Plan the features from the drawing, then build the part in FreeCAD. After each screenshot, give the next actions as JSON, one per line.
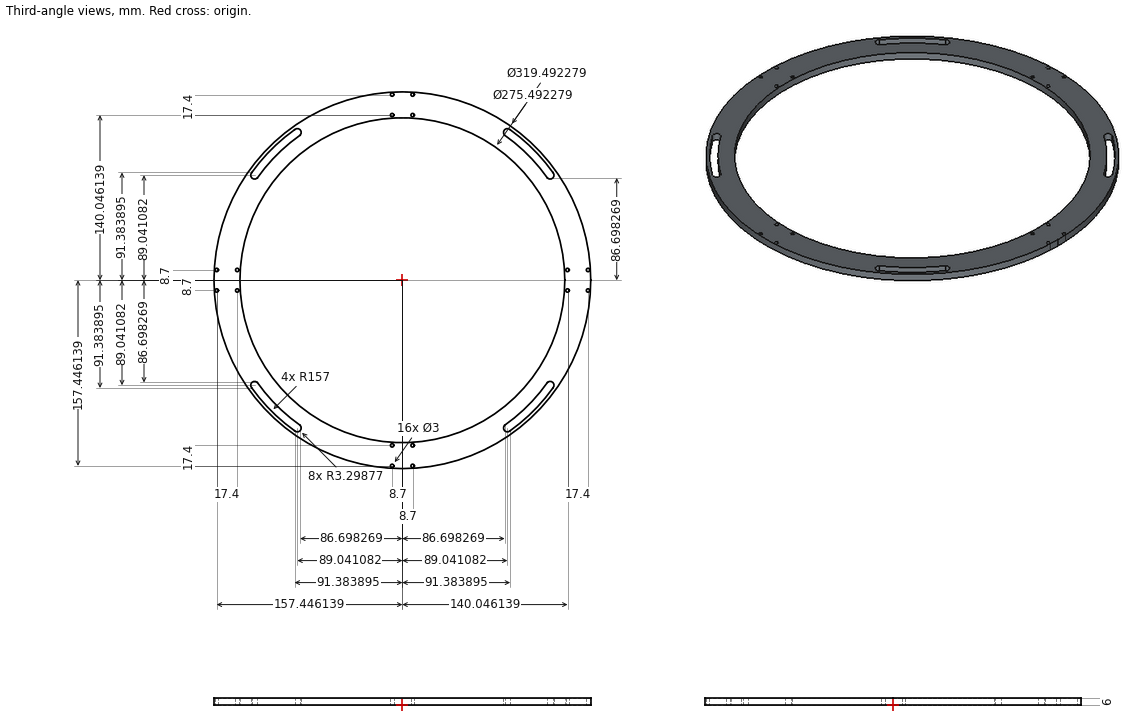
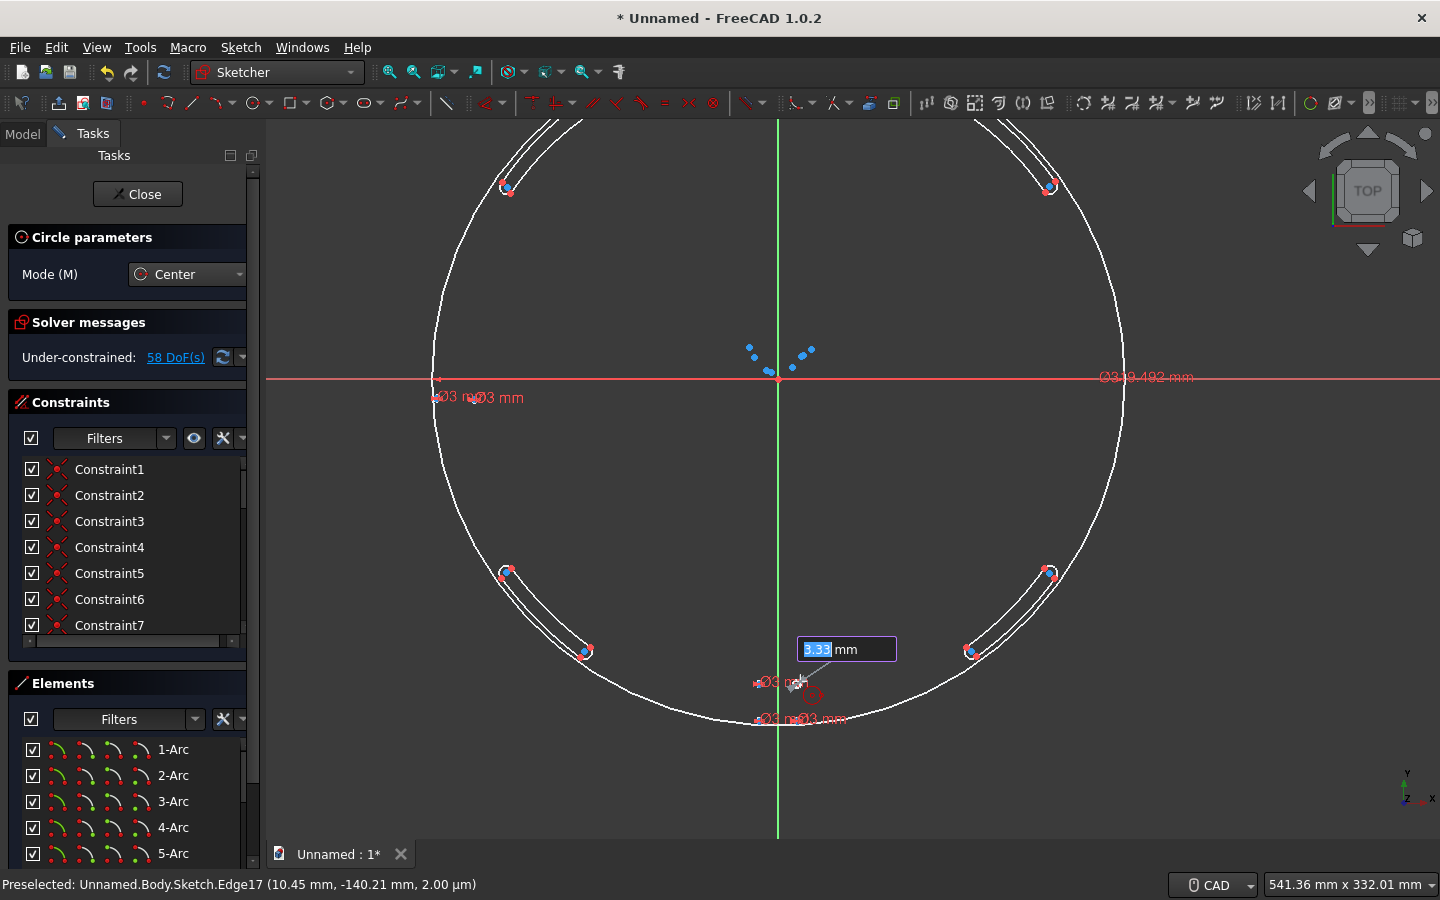
{"action": "type", "text": "3"}
{"action": "key", "text": "Return"}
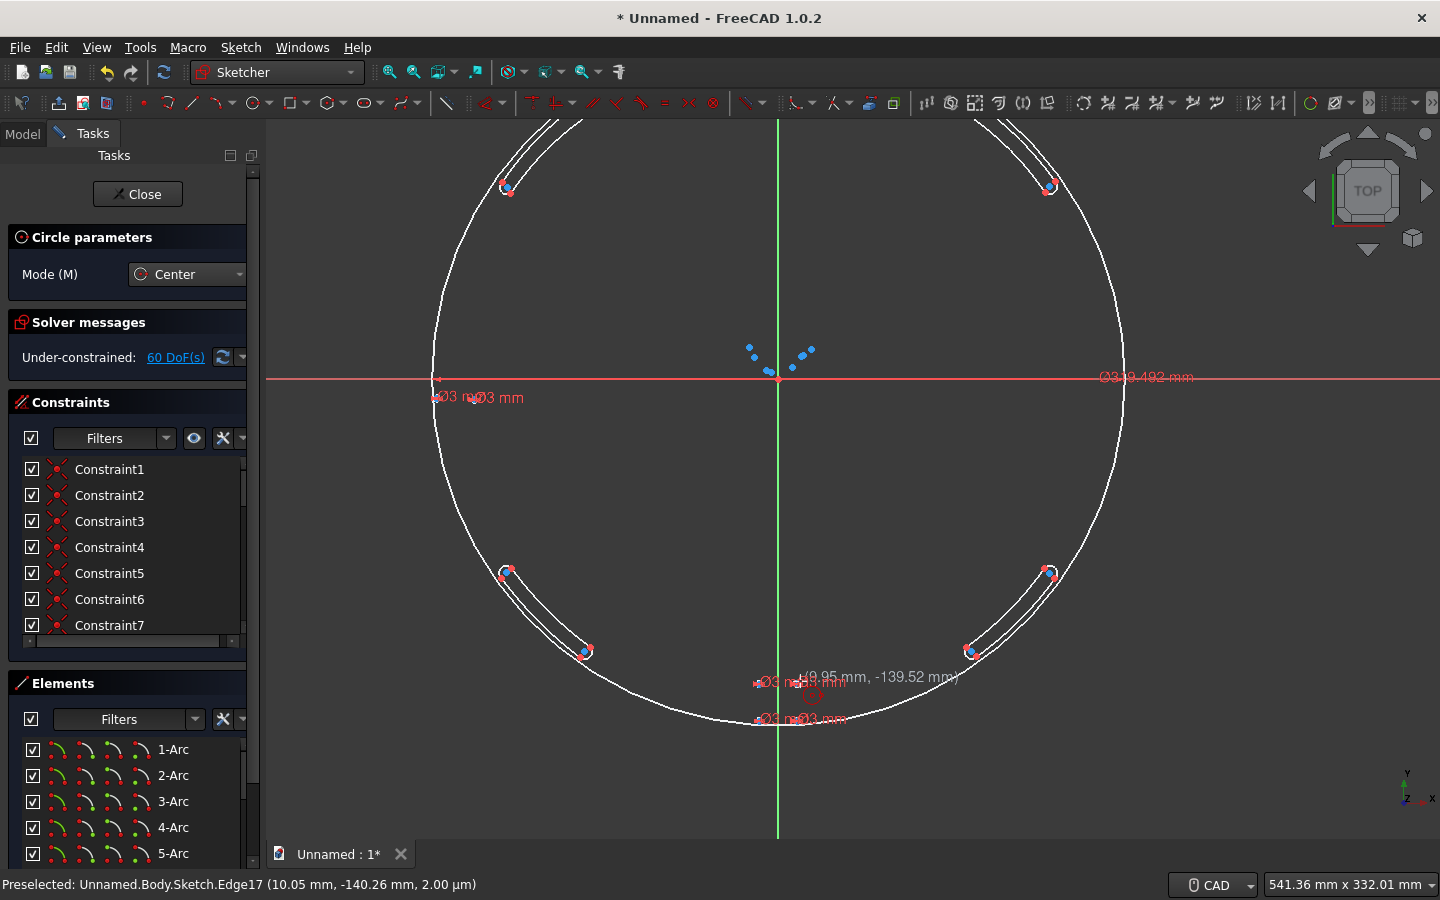
{"action": "scroll", "coordinate": [1082, 398], "scroll_direction": "up", "scroll_amount": 10}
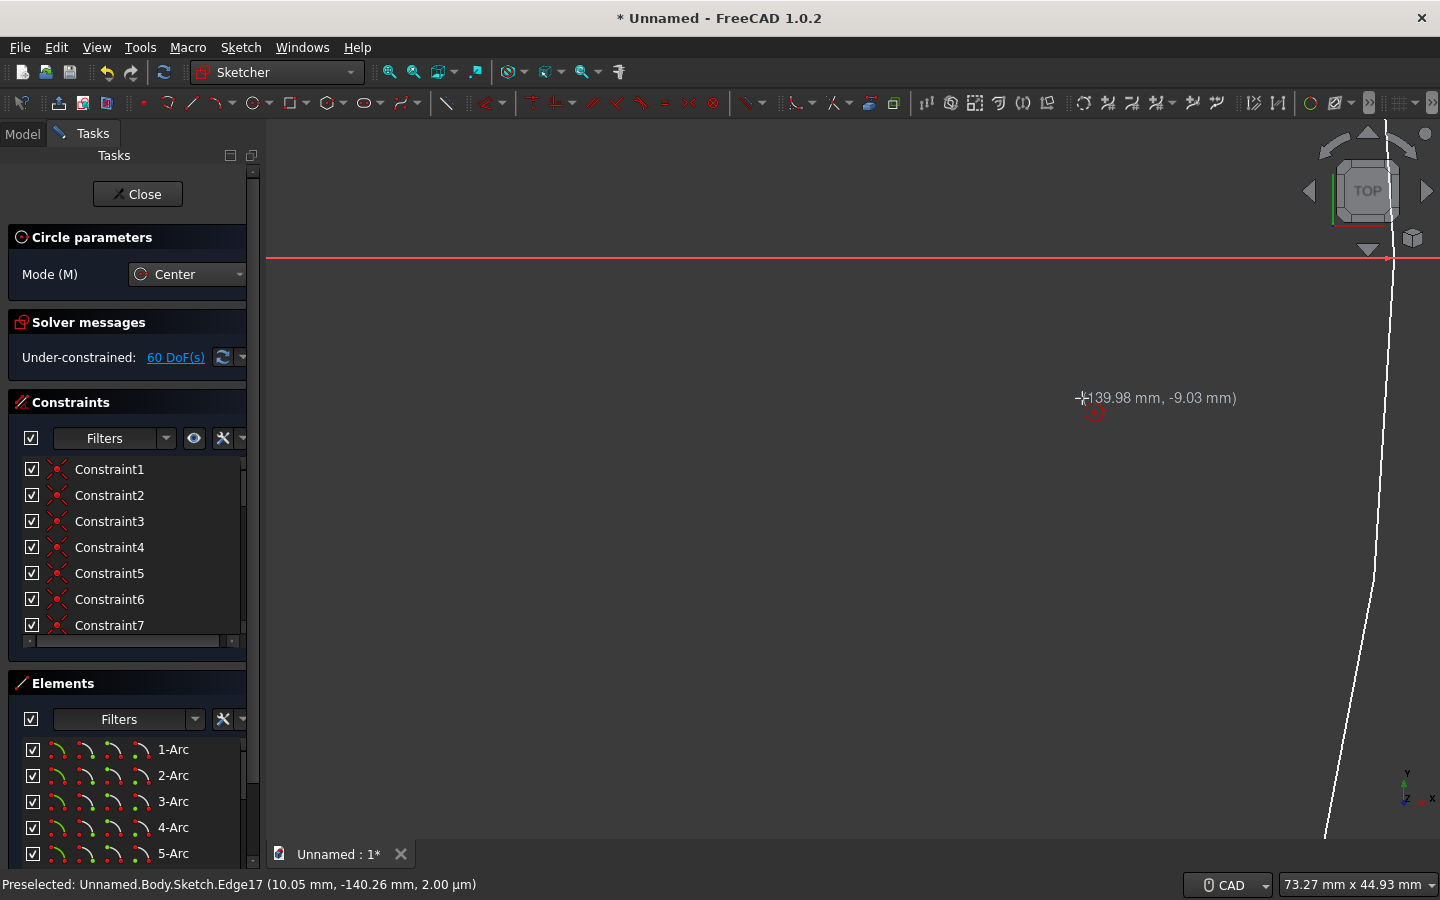
{"action": "scroll", "coordinate": [979, 501], "scroll_direction": "down", "scroll_amount": 12}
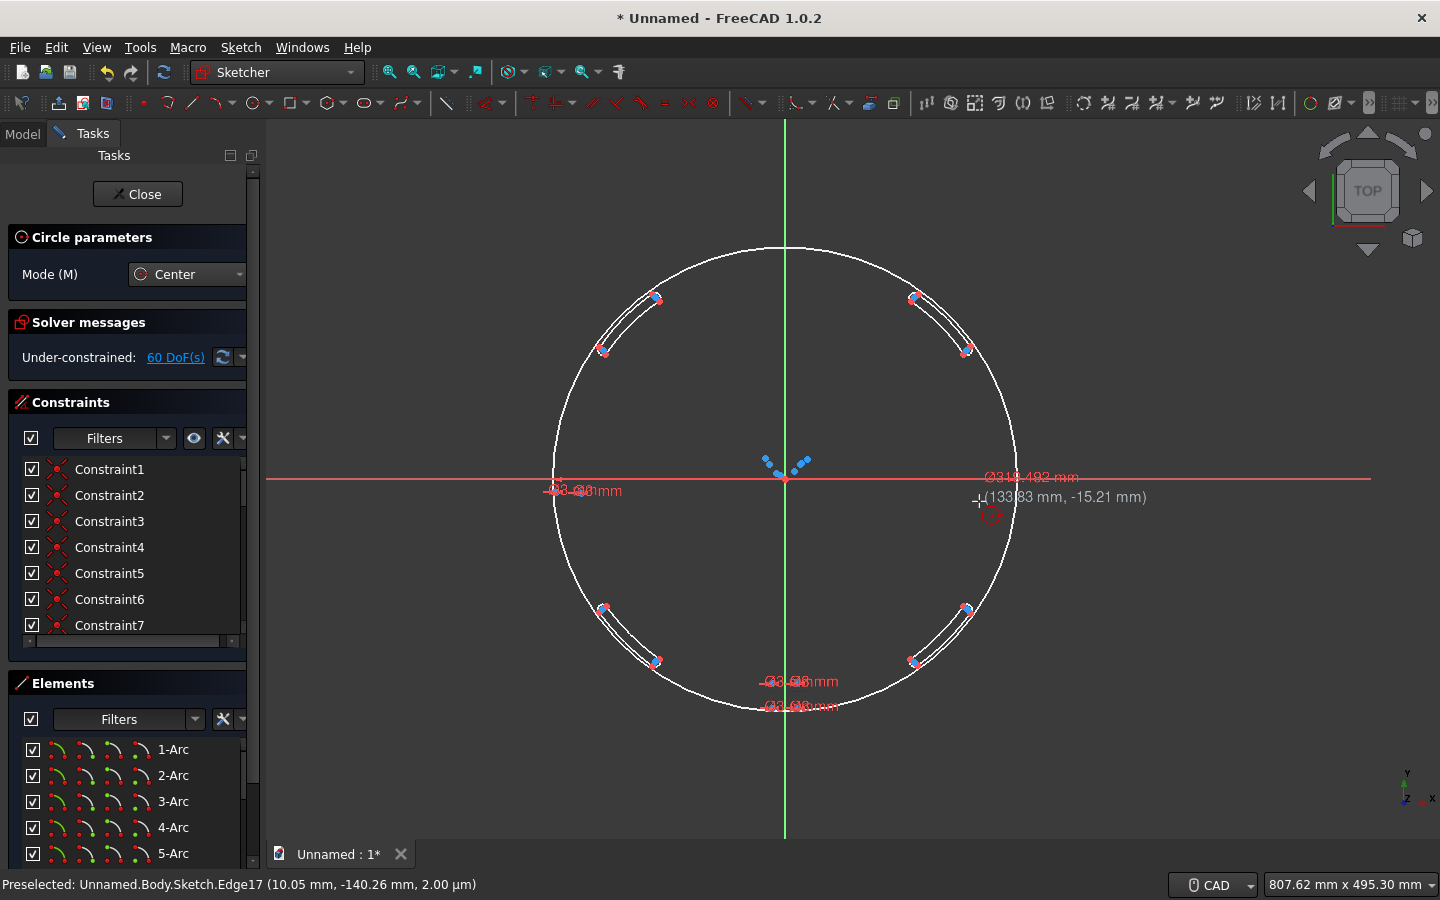
{"action": "scroll", "coordinate": [989, 492], "scroll_direction": "up", "scroll_amount": 2}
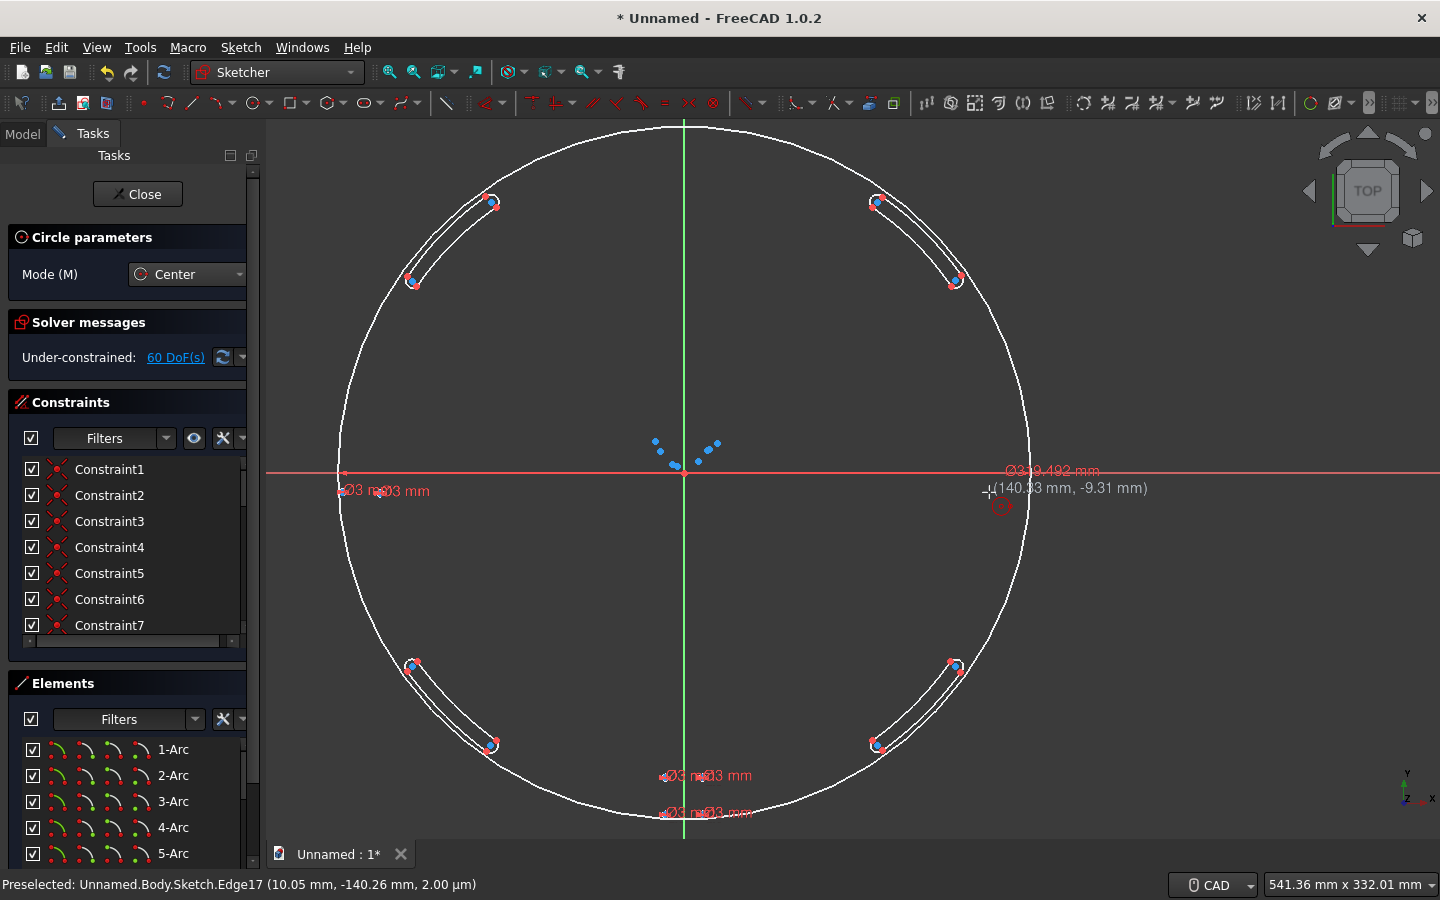
{"action": "left_click", "coordinate": [988, 492]}
{"action": "mouse_move", "coordinate": [990, 490]}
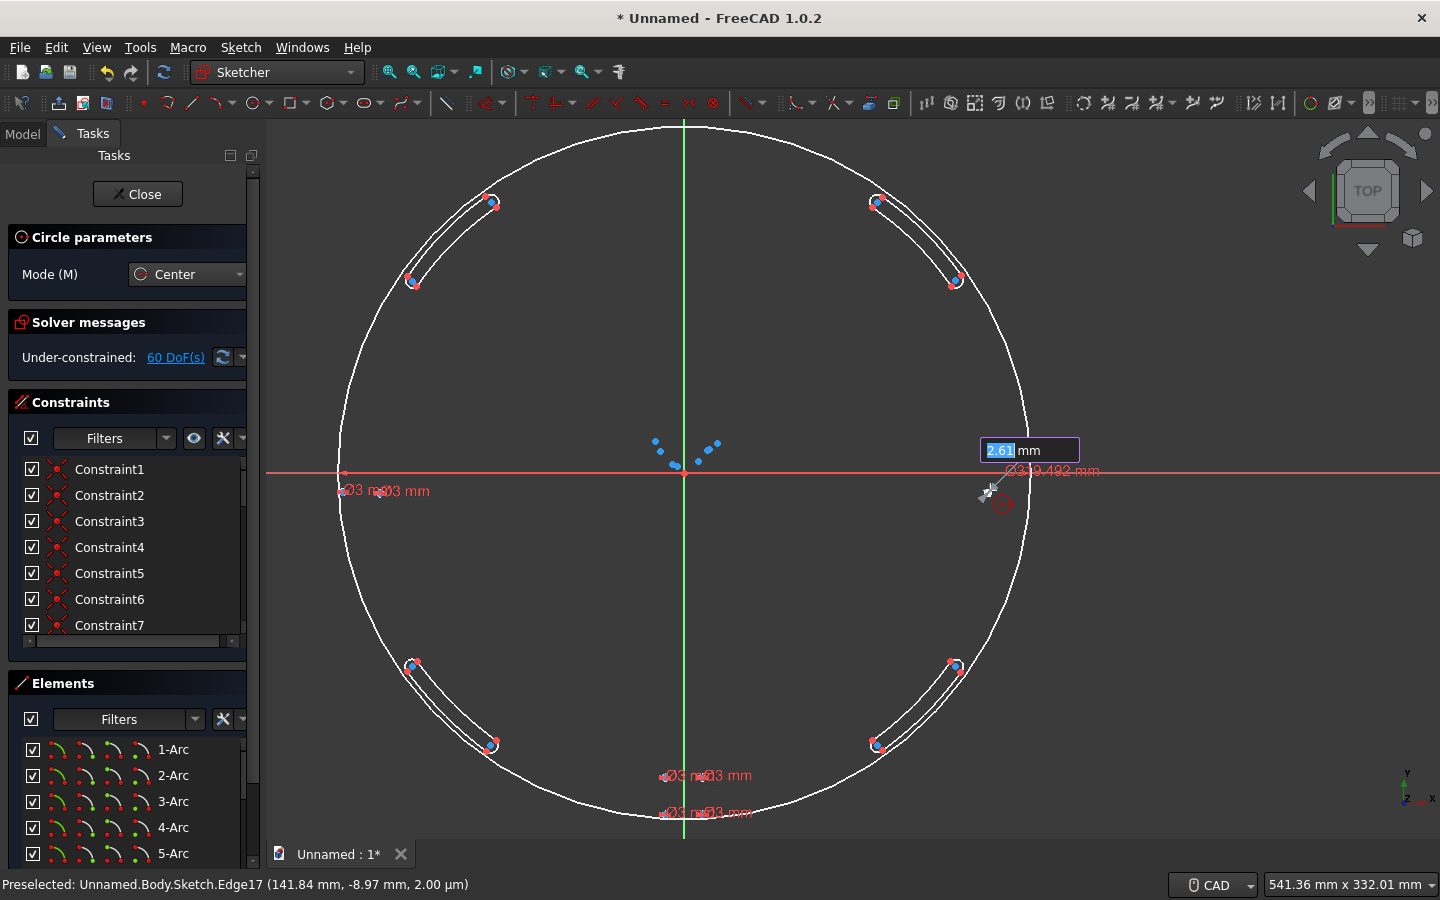
{"action": "type", "text": "3"}
{"action": "key", "text": "Return"}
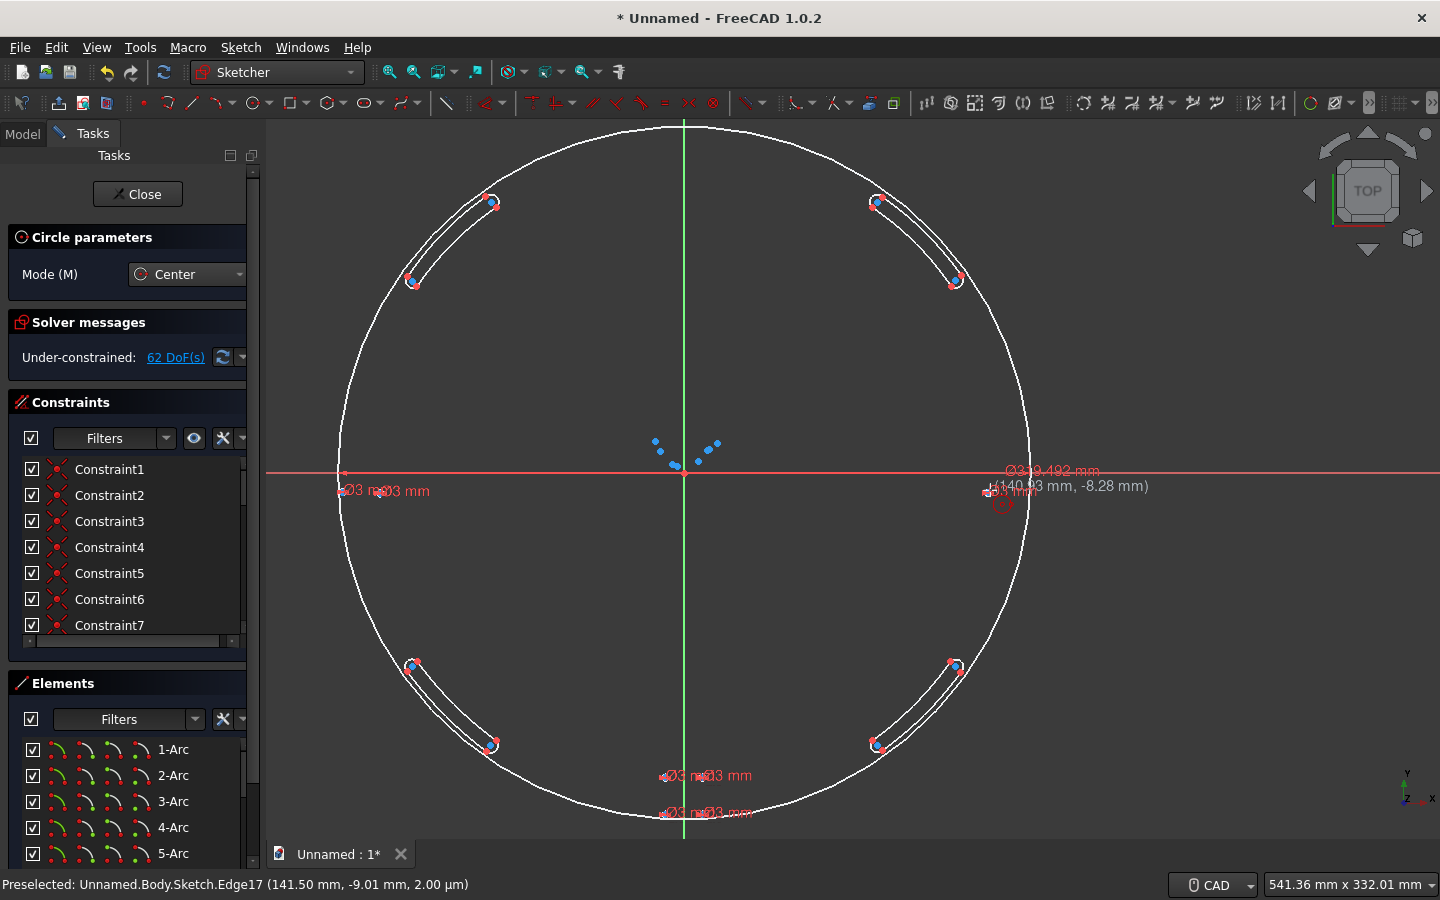
{"action": "scroll", "coordinate": [1026, 492], "scroll_direction": "up", "scroll_amount": 10}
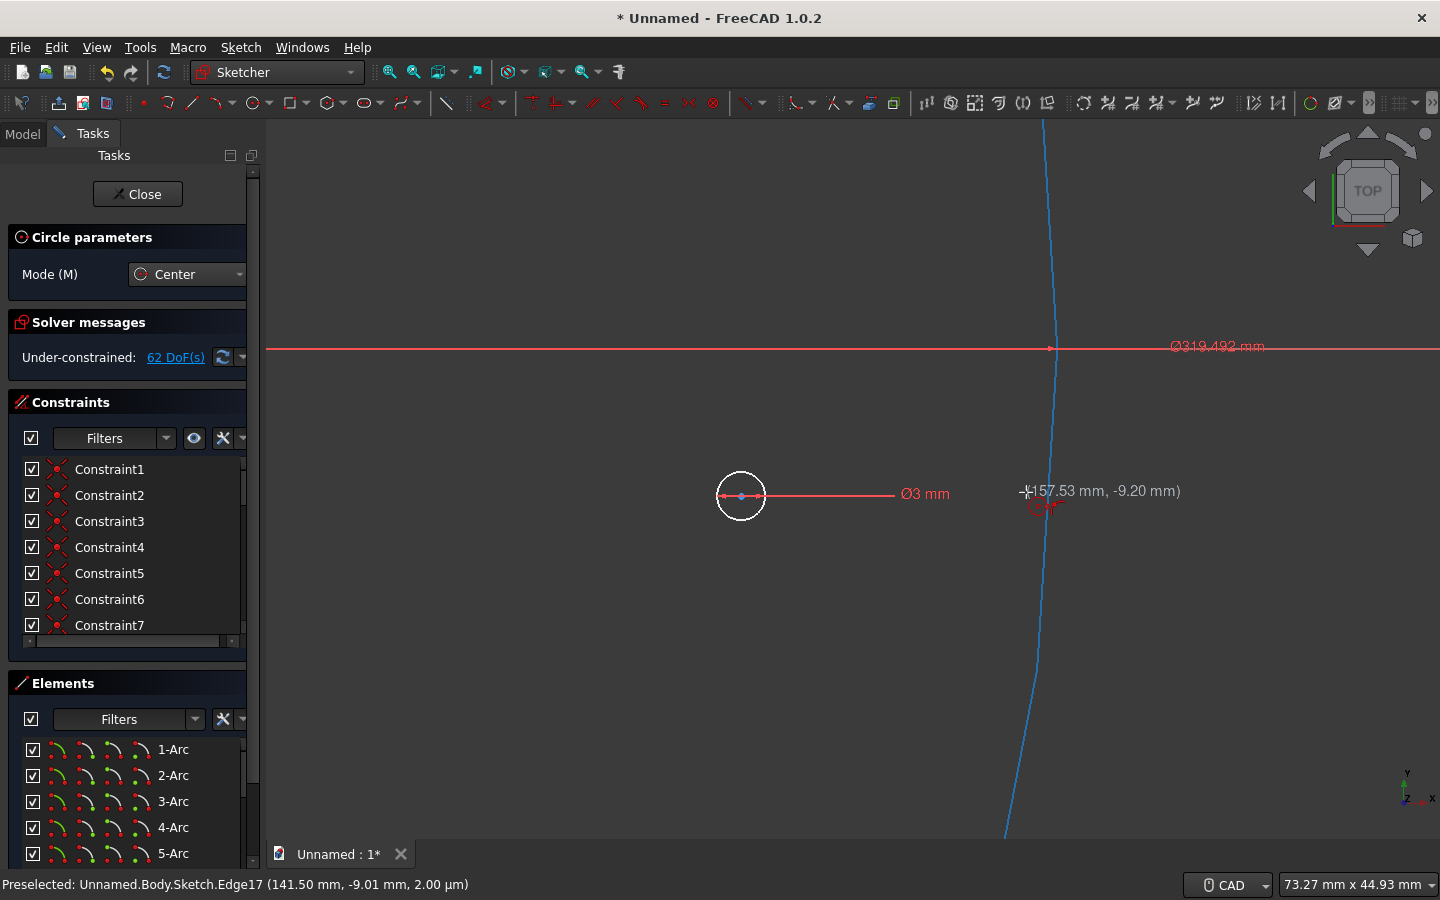
{"action": "left_click", "coordinate": [1020, 488]}
{"action": "mouse_move", "coordinate": [1037, 471]}